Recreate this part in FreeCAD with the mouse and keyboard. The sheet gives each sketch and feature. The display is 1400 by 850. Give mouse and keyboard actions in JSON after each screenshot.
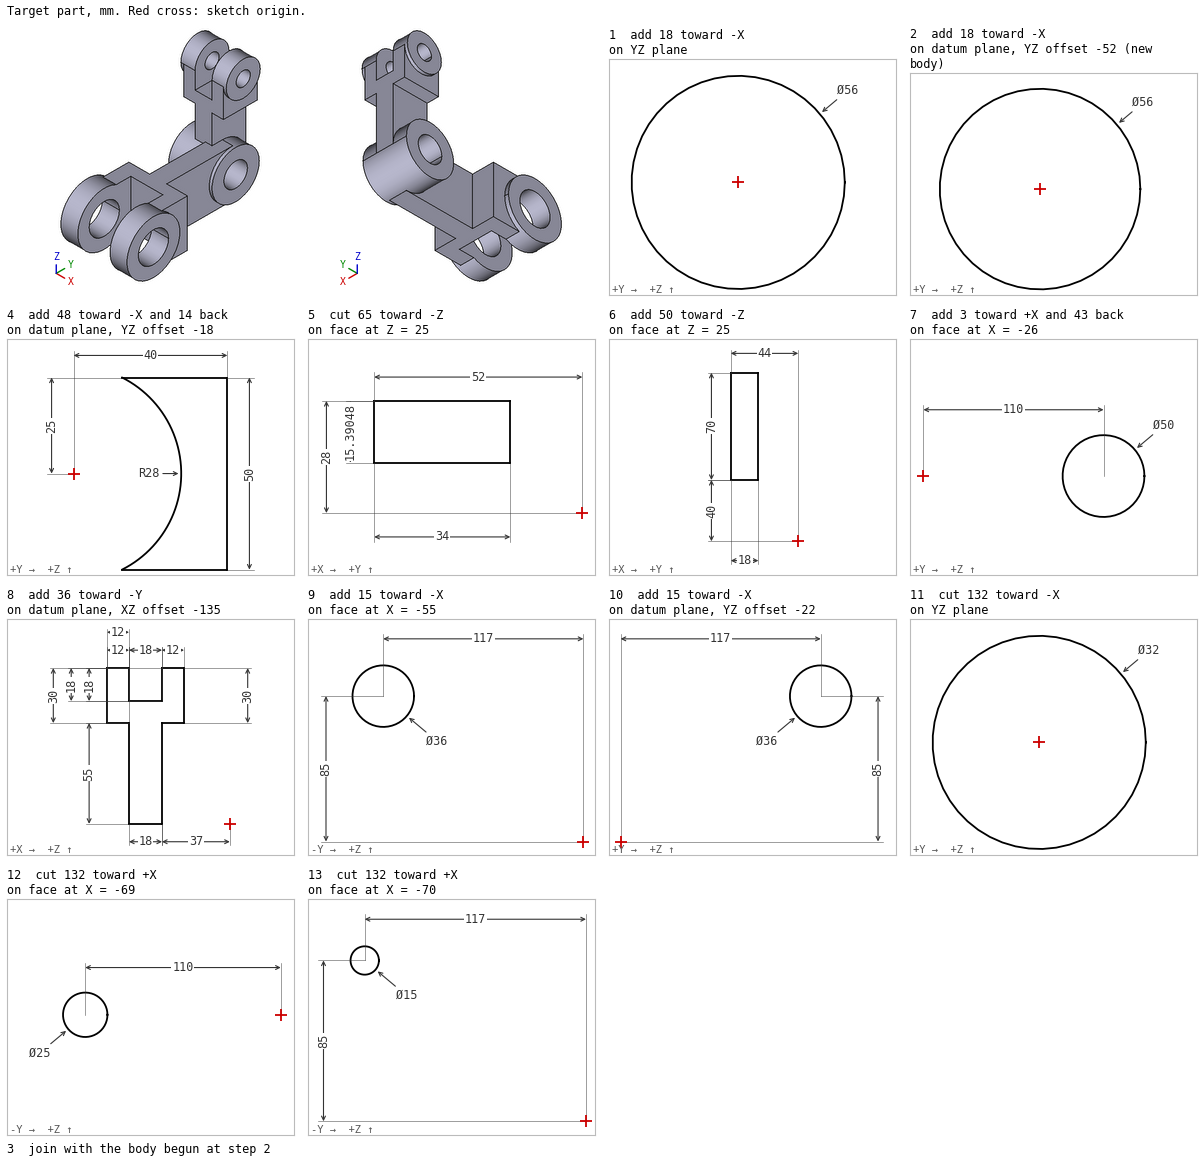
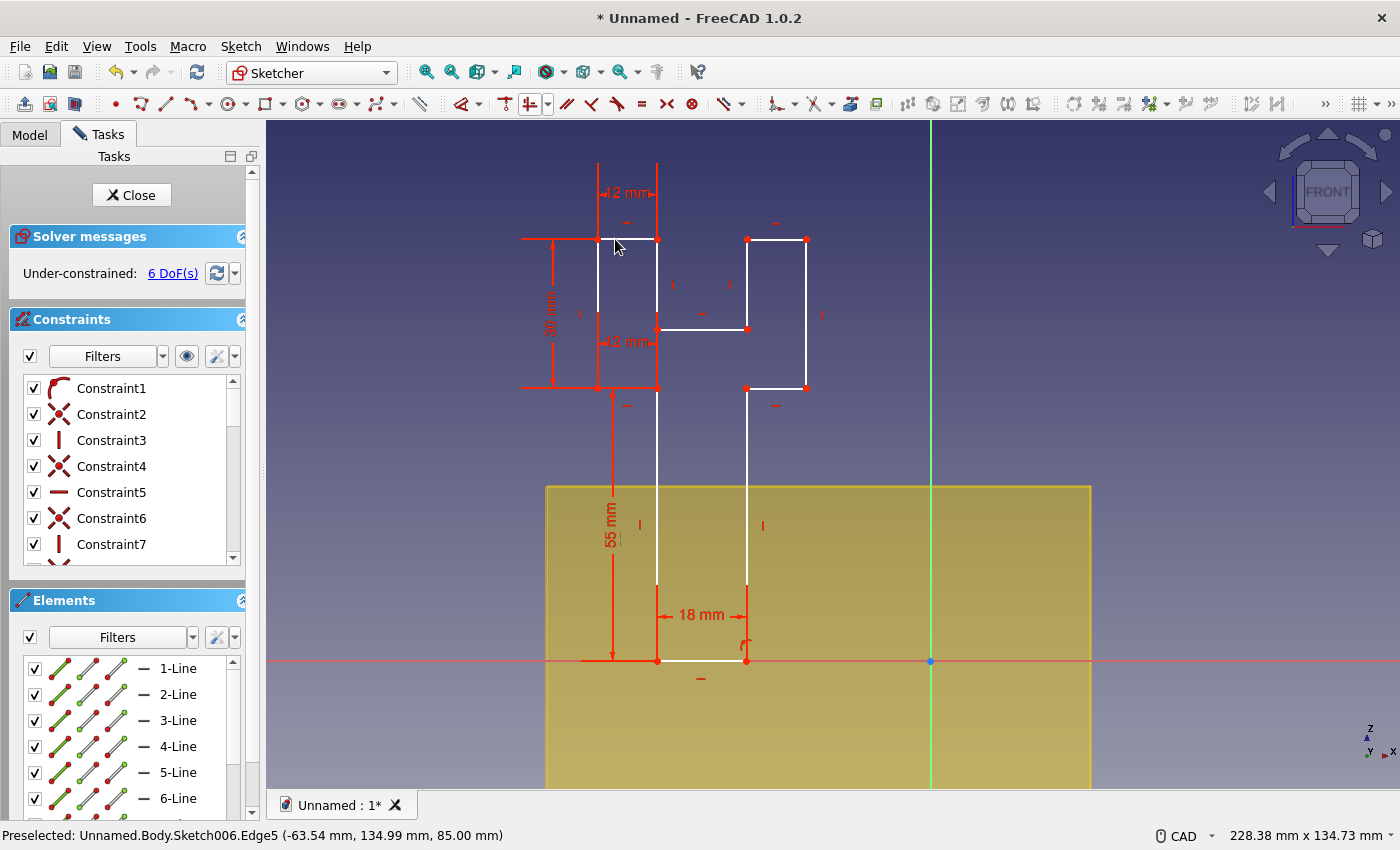
{"action": "left_click", "coordinate": [657, 267]}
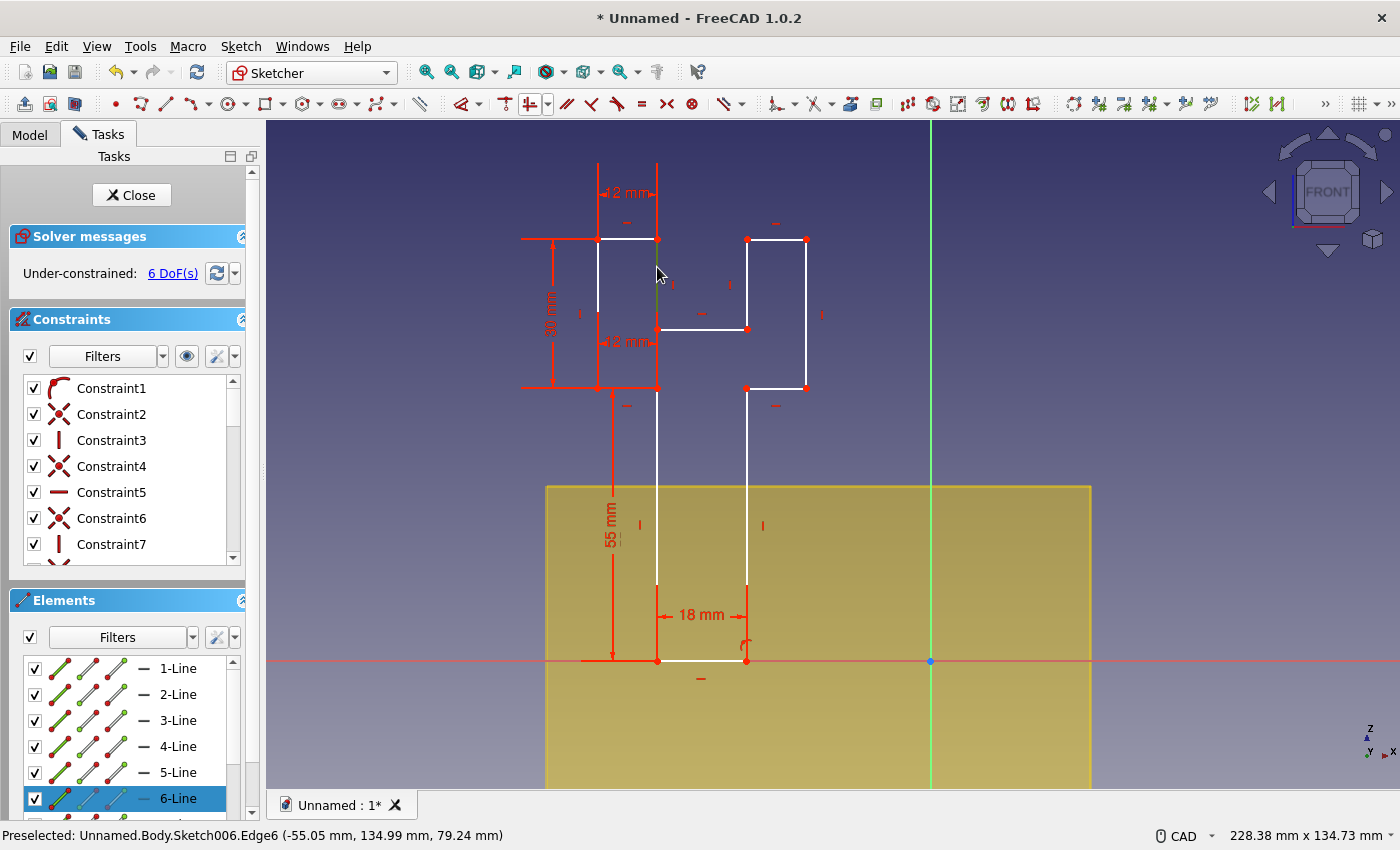
{"action": "left_click", "coordinate": [478, 104]}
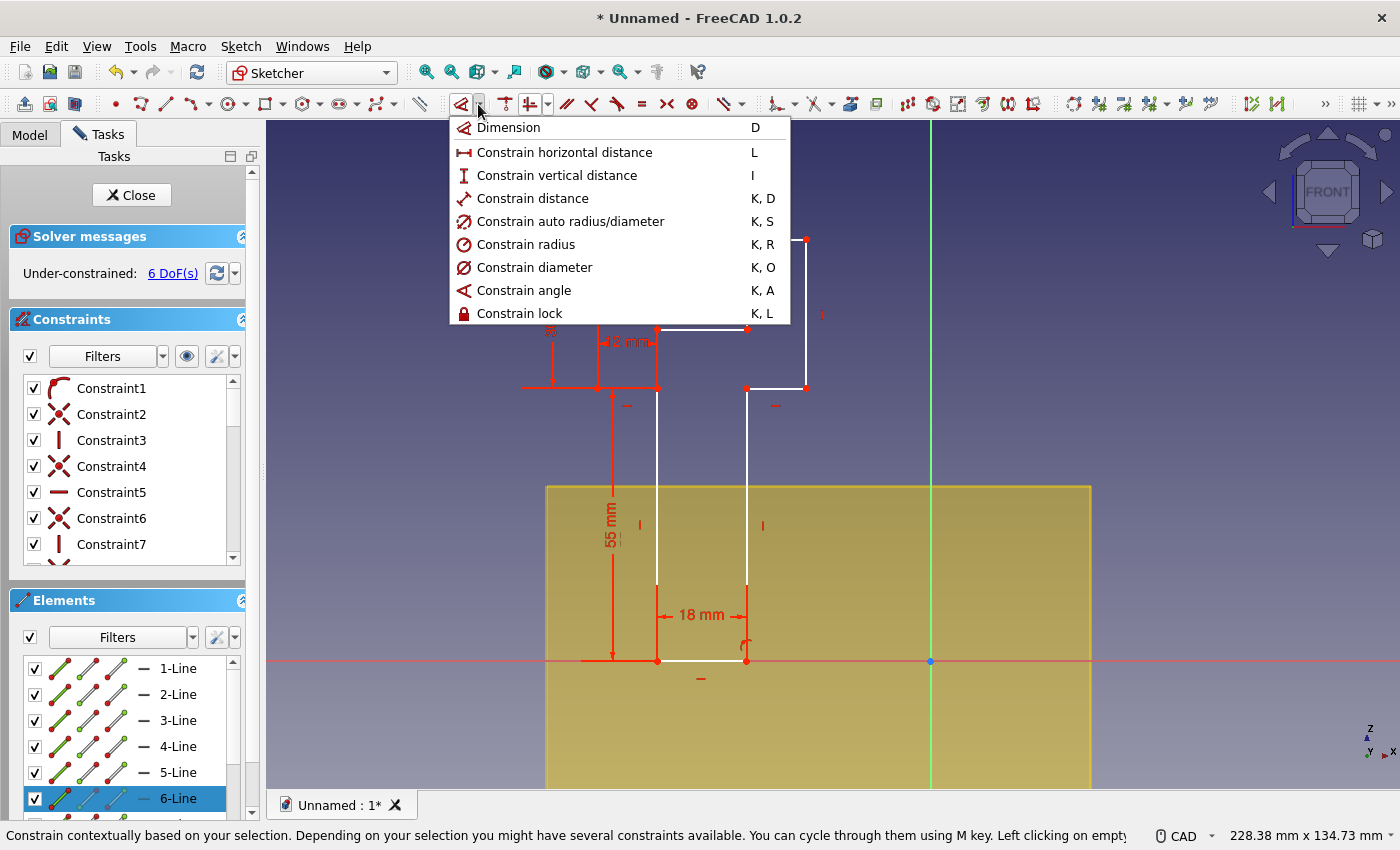
{"action": "left_click", "coordinate": [620, 176]}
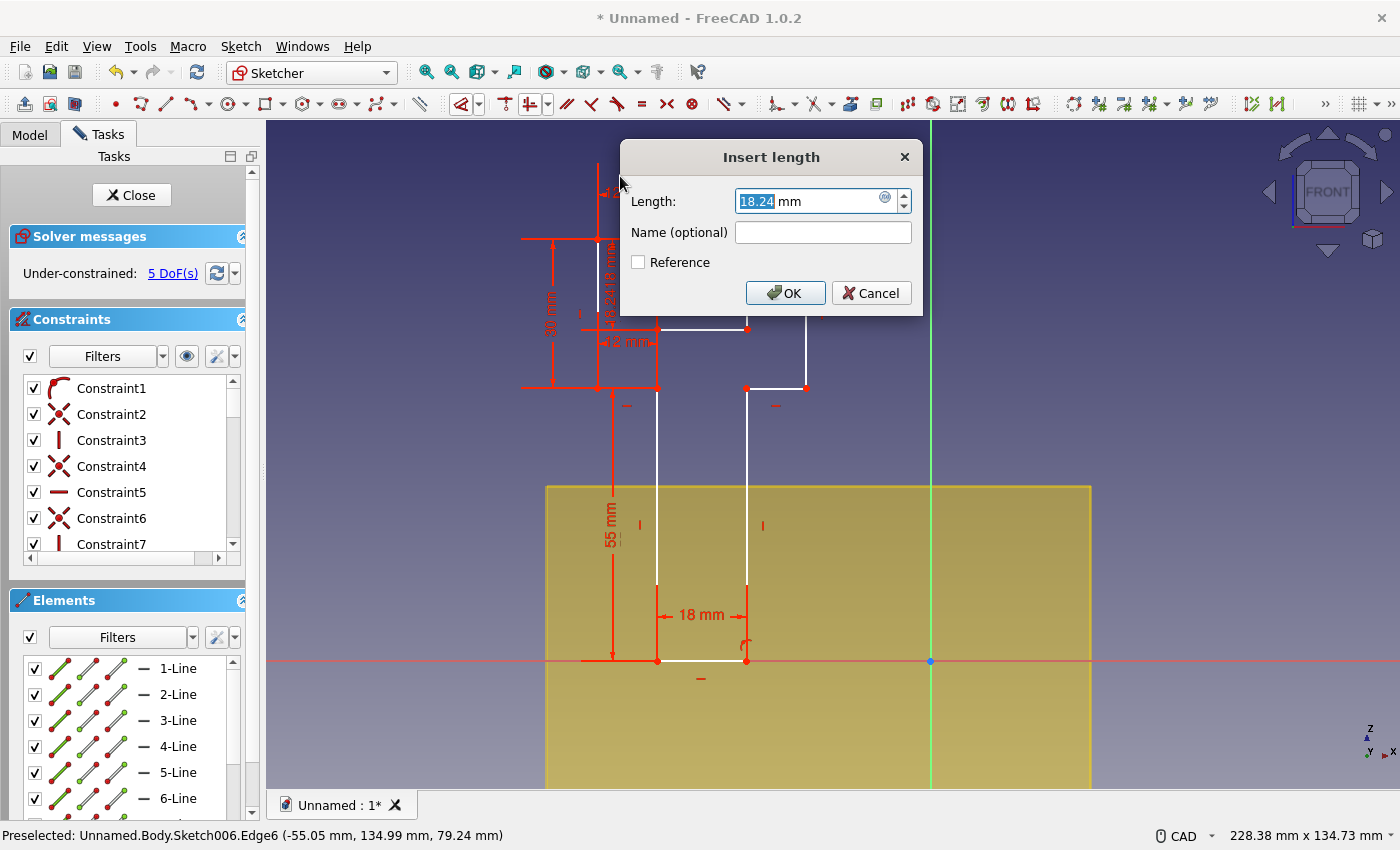
{"action": "type", "text": "18"}
{"action": "key", "text": "Return"}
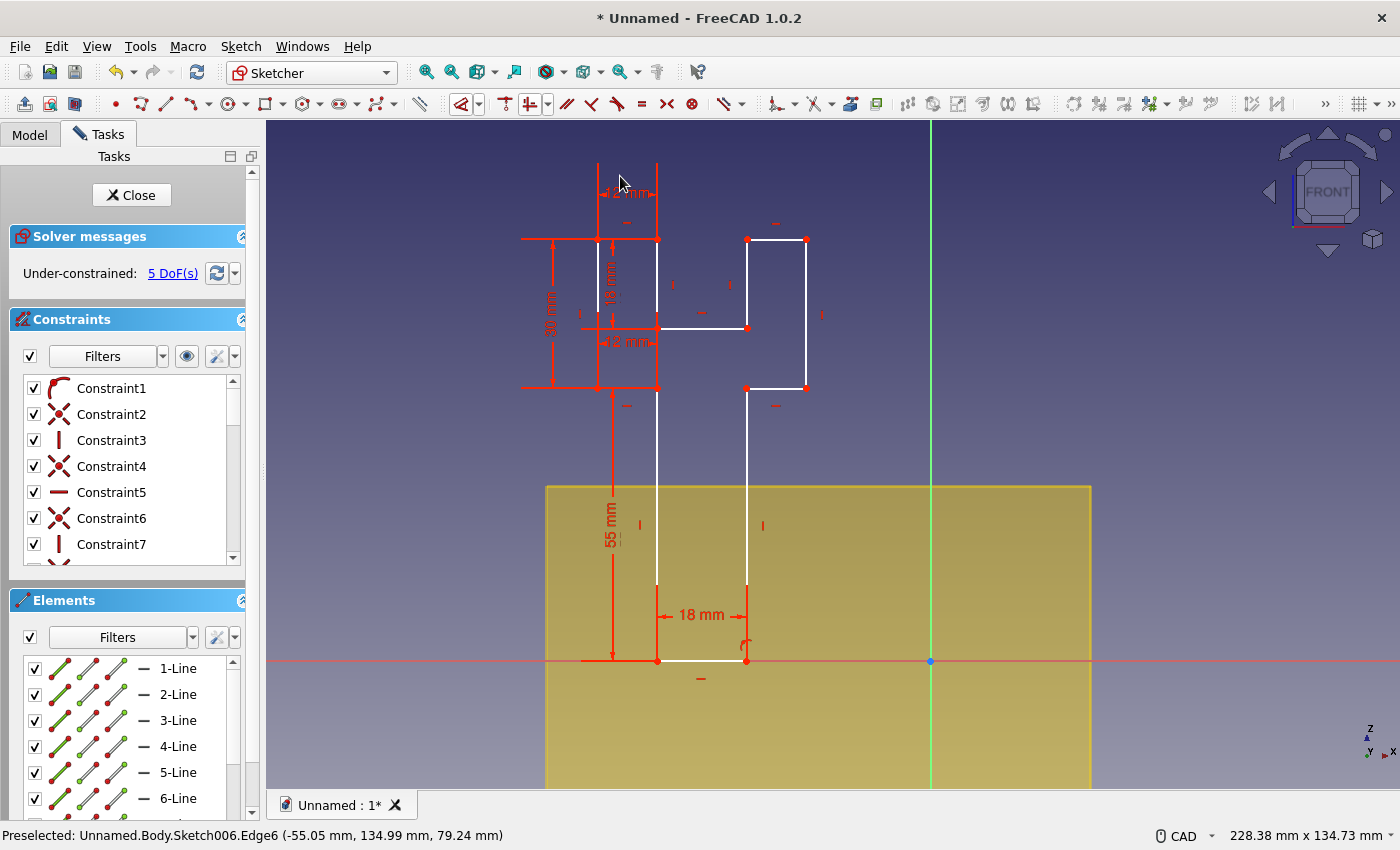
{"action": "left_click", "coordinate": [684, 329]}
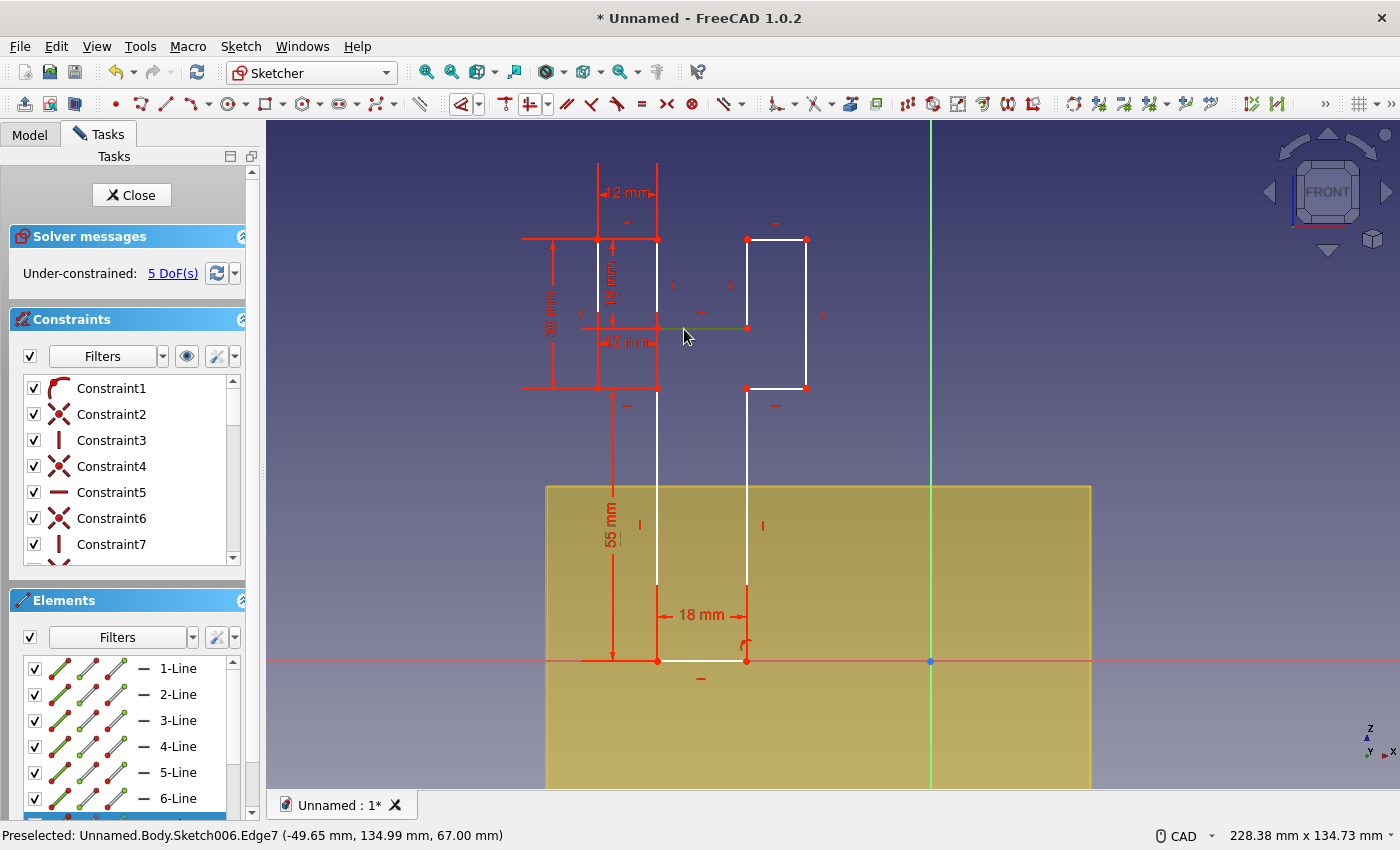
{"action": "left_click", "coordinate": [478, 104]}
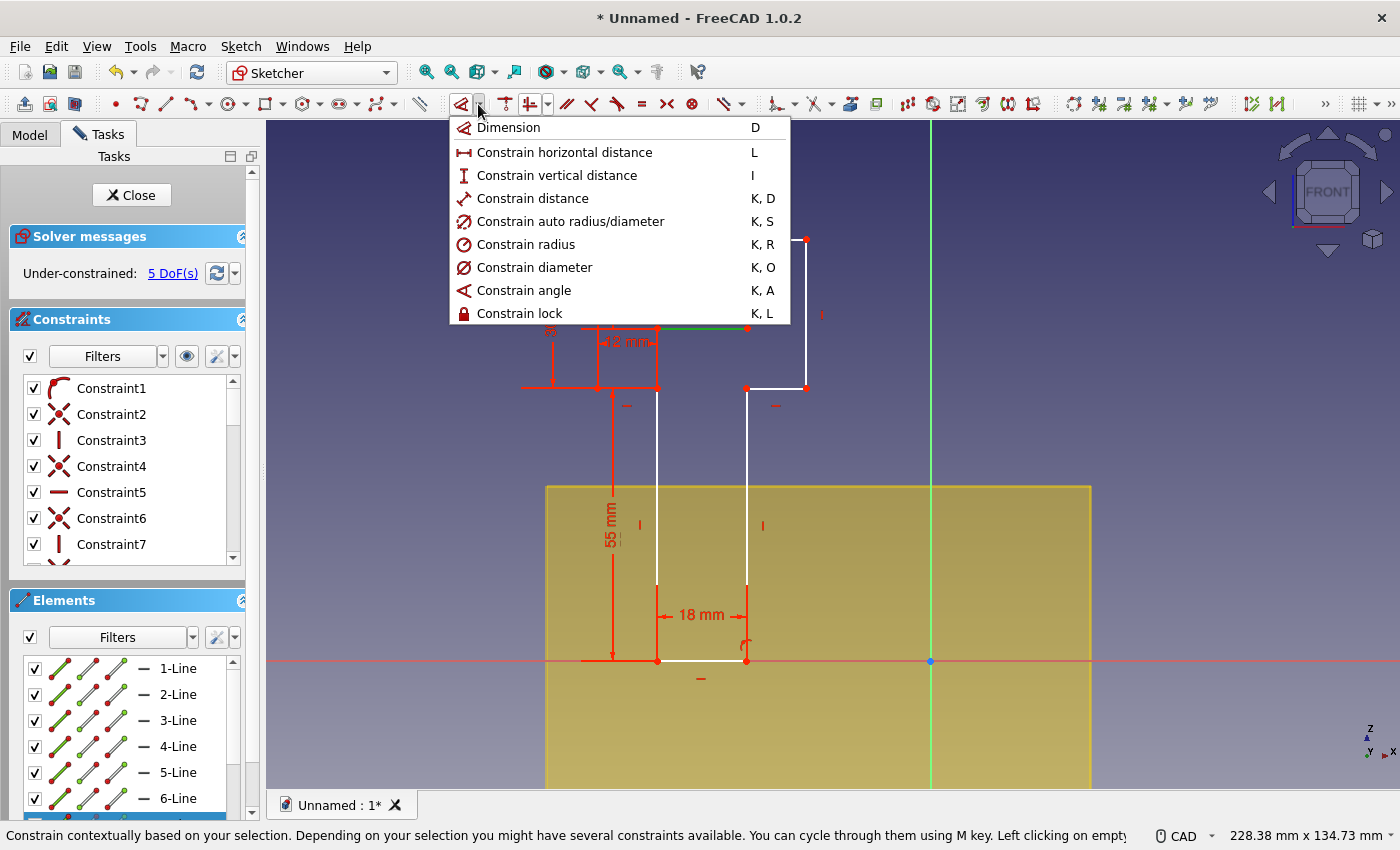
{"action": "left_click", "coordinate": [620, 152]}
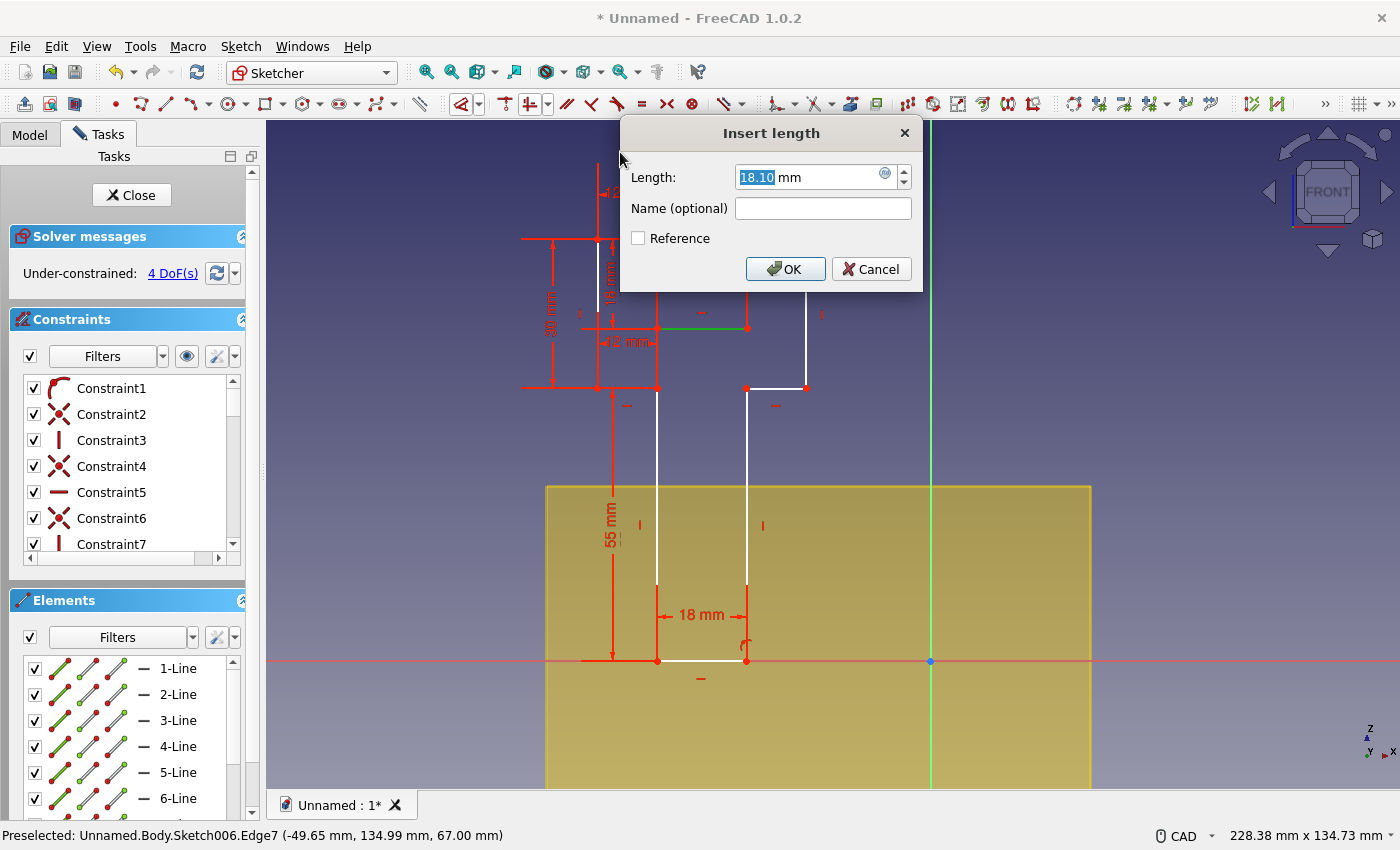
{"action": "type", "text": "18"}
{"action": "key", "text": "Return"}